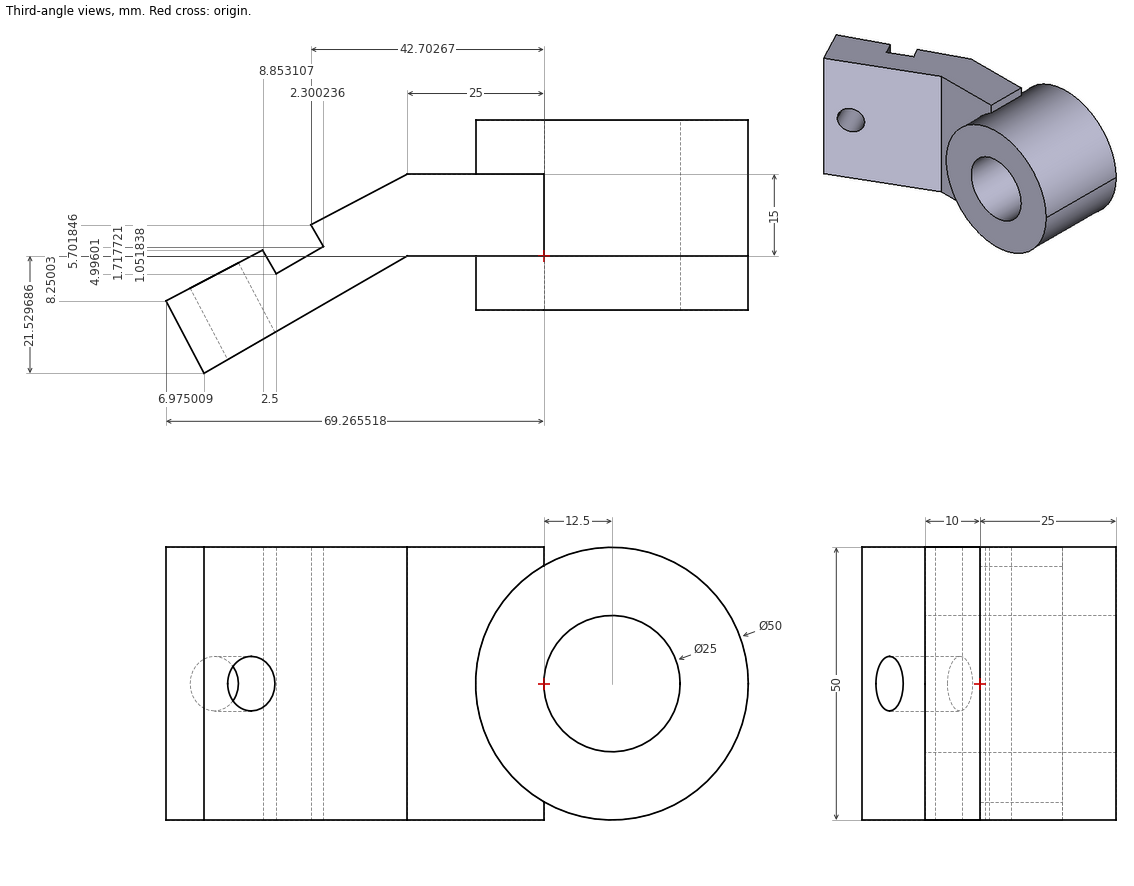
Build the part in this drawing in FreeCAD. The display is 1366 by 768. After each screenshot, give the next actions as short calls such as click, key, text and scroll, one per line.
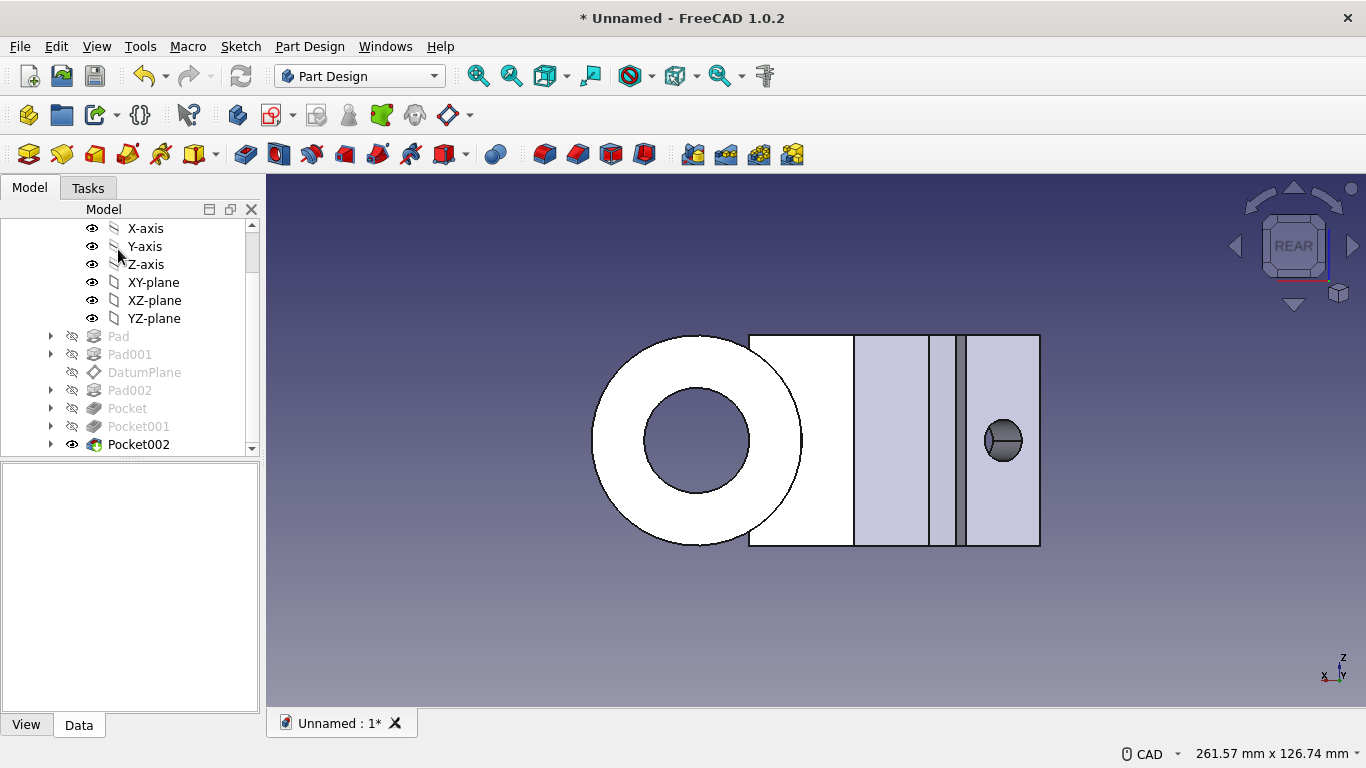
key(0)